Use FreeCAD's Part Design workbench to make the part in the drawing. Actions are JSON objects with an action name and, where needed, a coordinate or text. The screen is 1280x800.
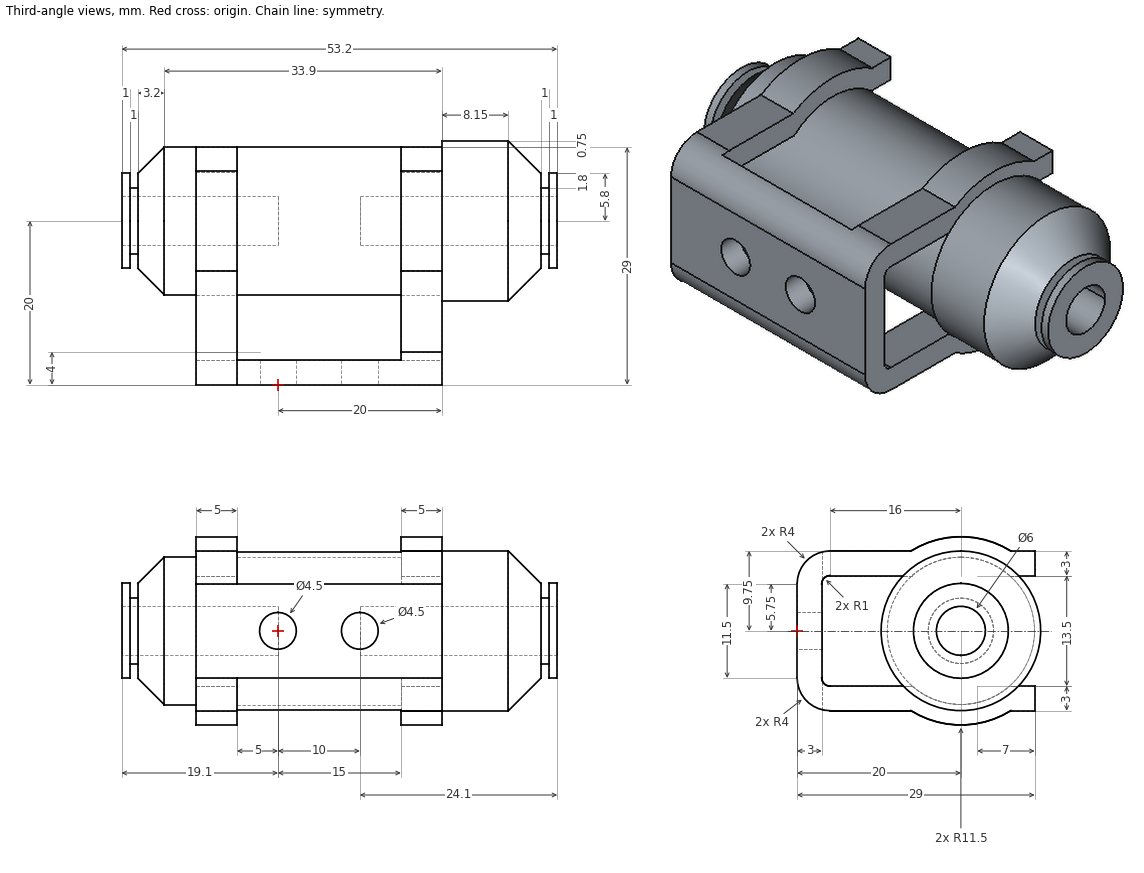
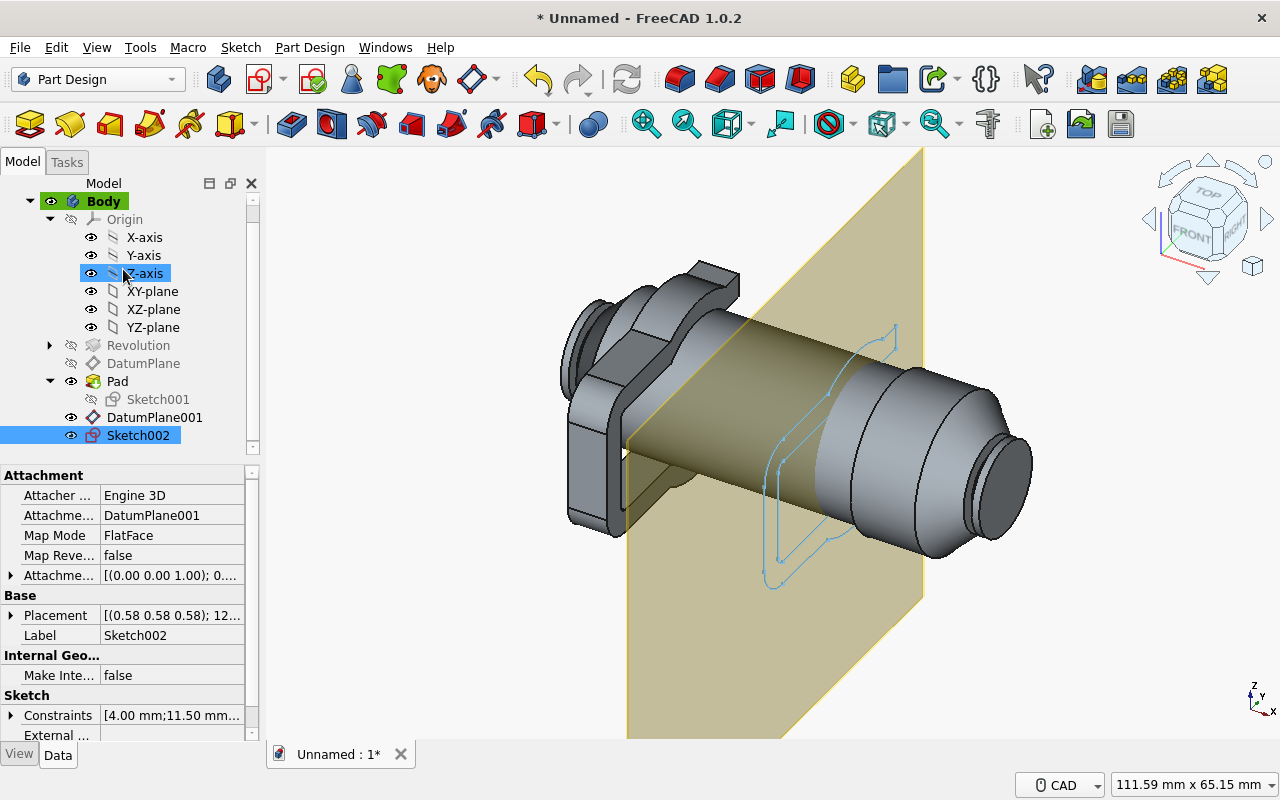
{"action": "left_click", "coordinate": [30, 124]}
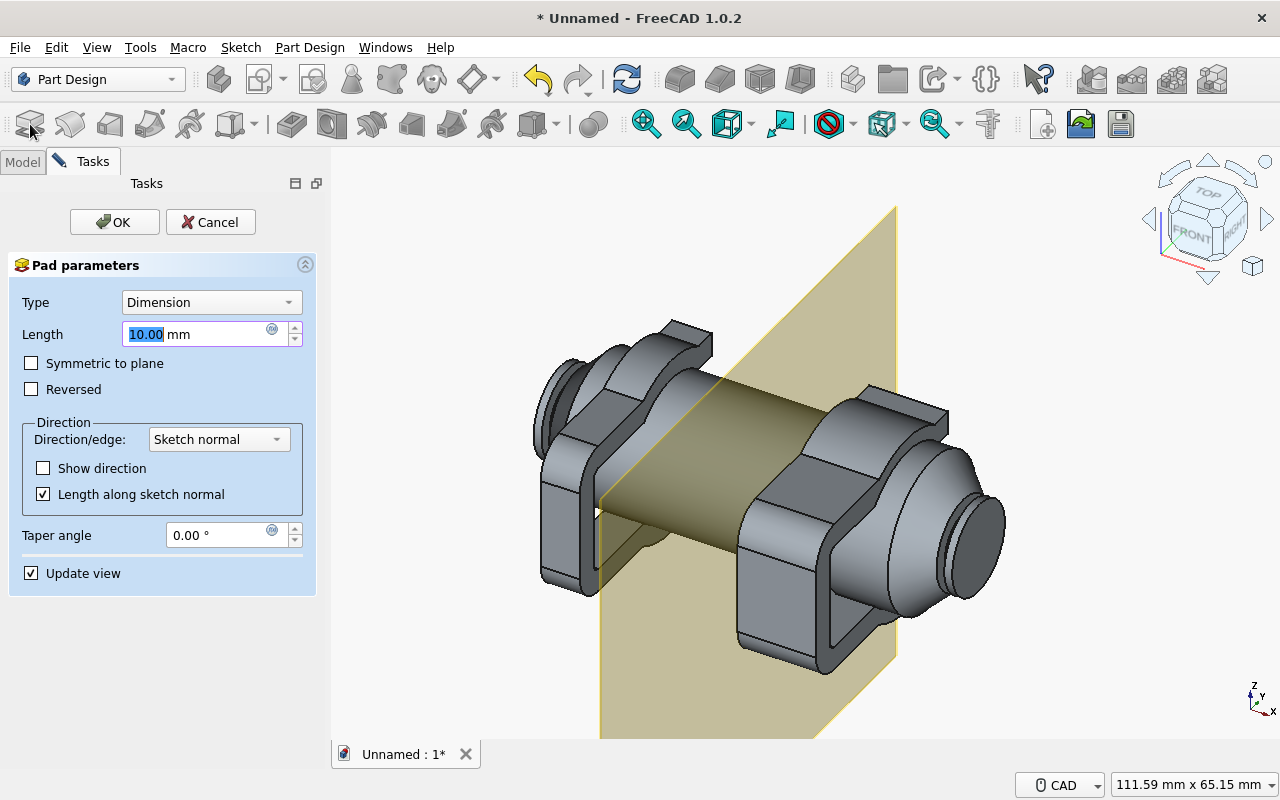
{"action": "type", "text": "5"}
{"action": "key", "text": "Tab"}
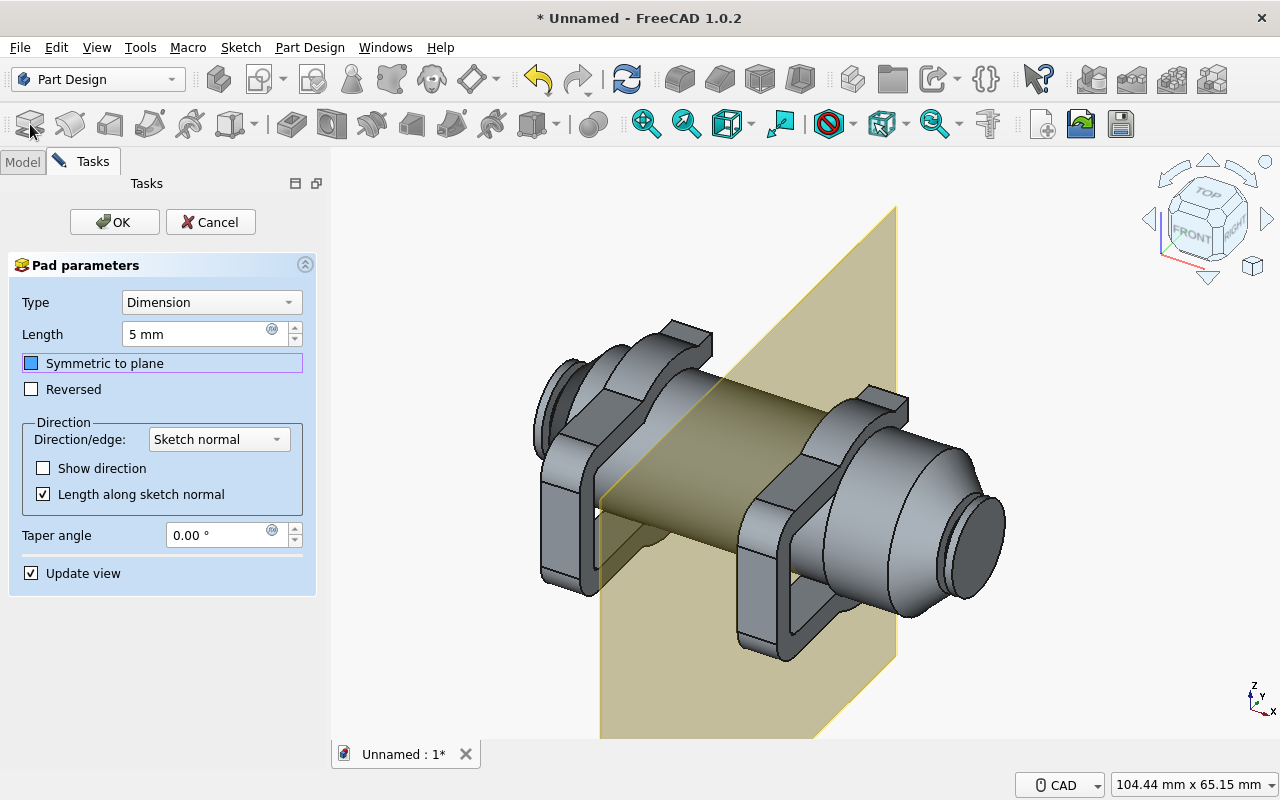
{"action": "left_click", "coordinate": [115, 222]}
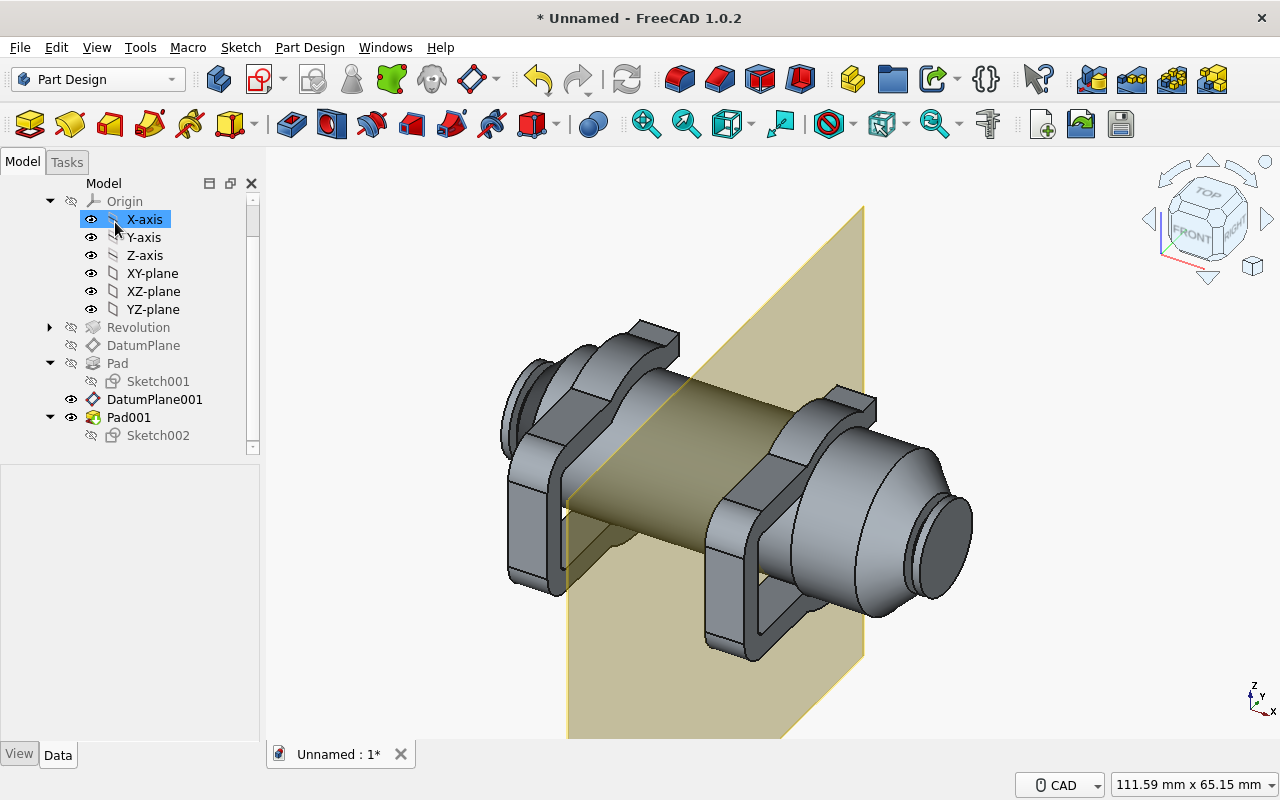
{"action": "left_click", "coordinate": [116, 399]}
{"action": "key", "text": "space"}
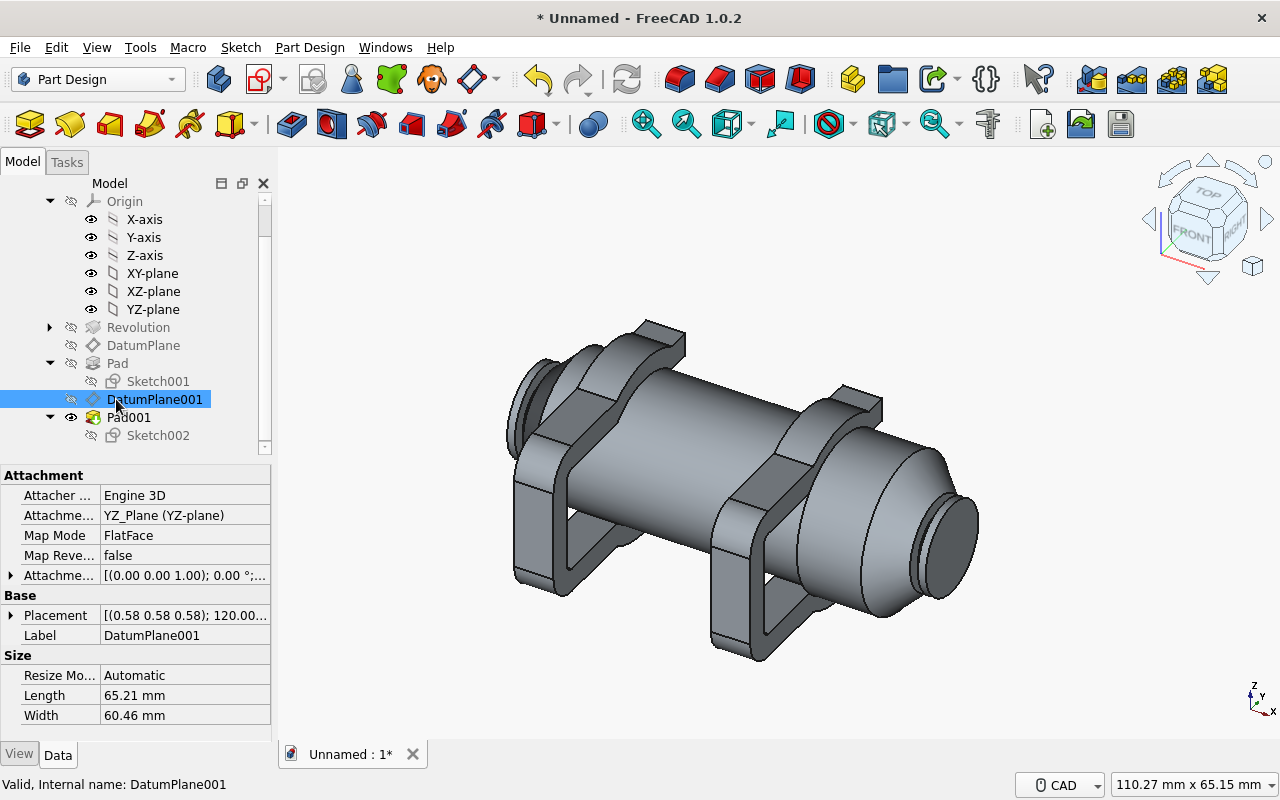
{"action": "left_click", "coordinate": [318, 699]}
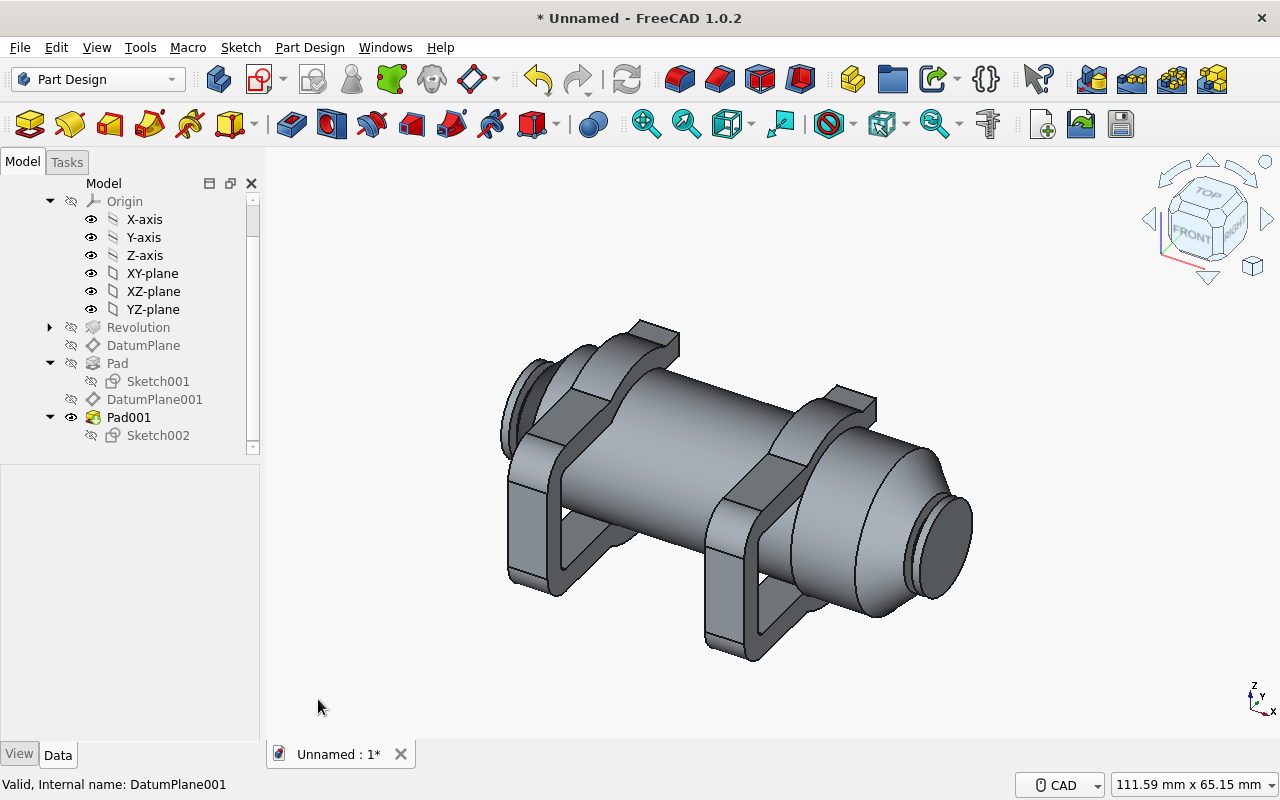
{"action": "left_click", "coordinate": [260, 80]}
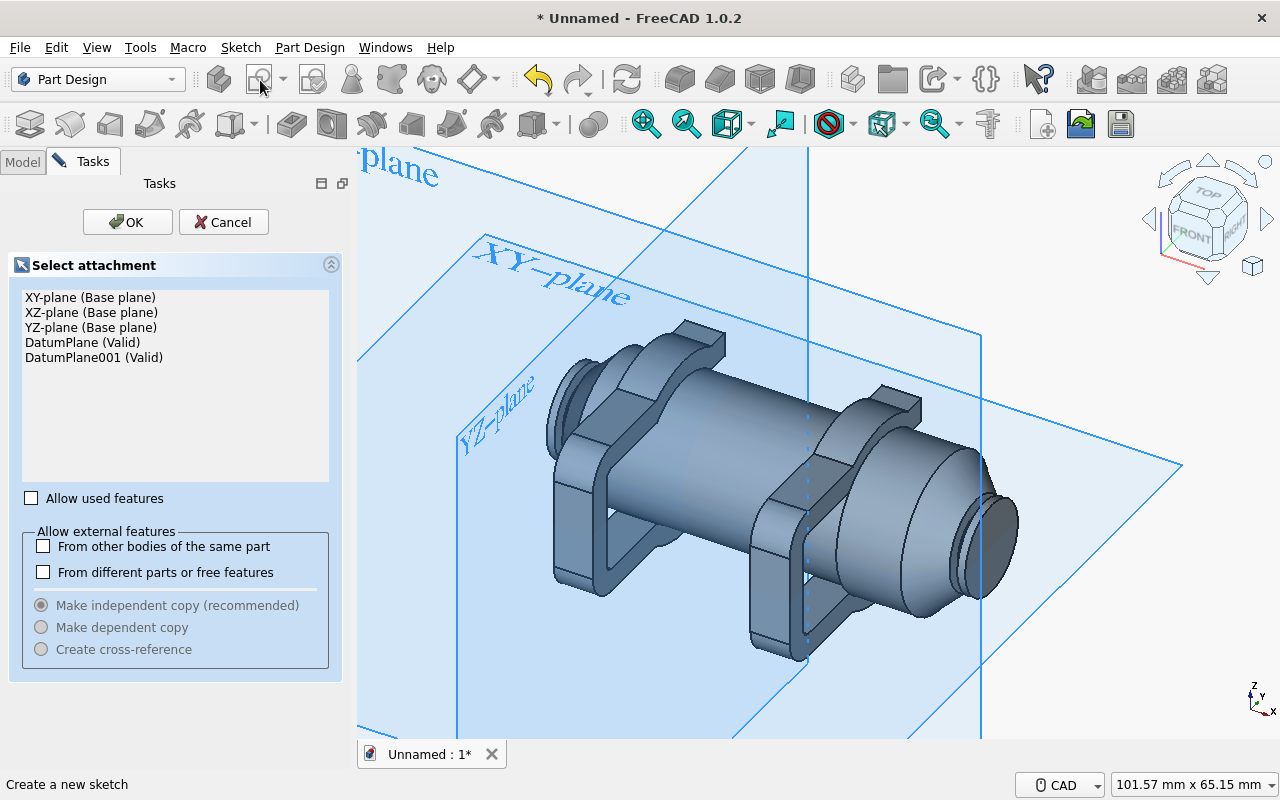
{"action": "left_click", "coordinate": [82, 328]}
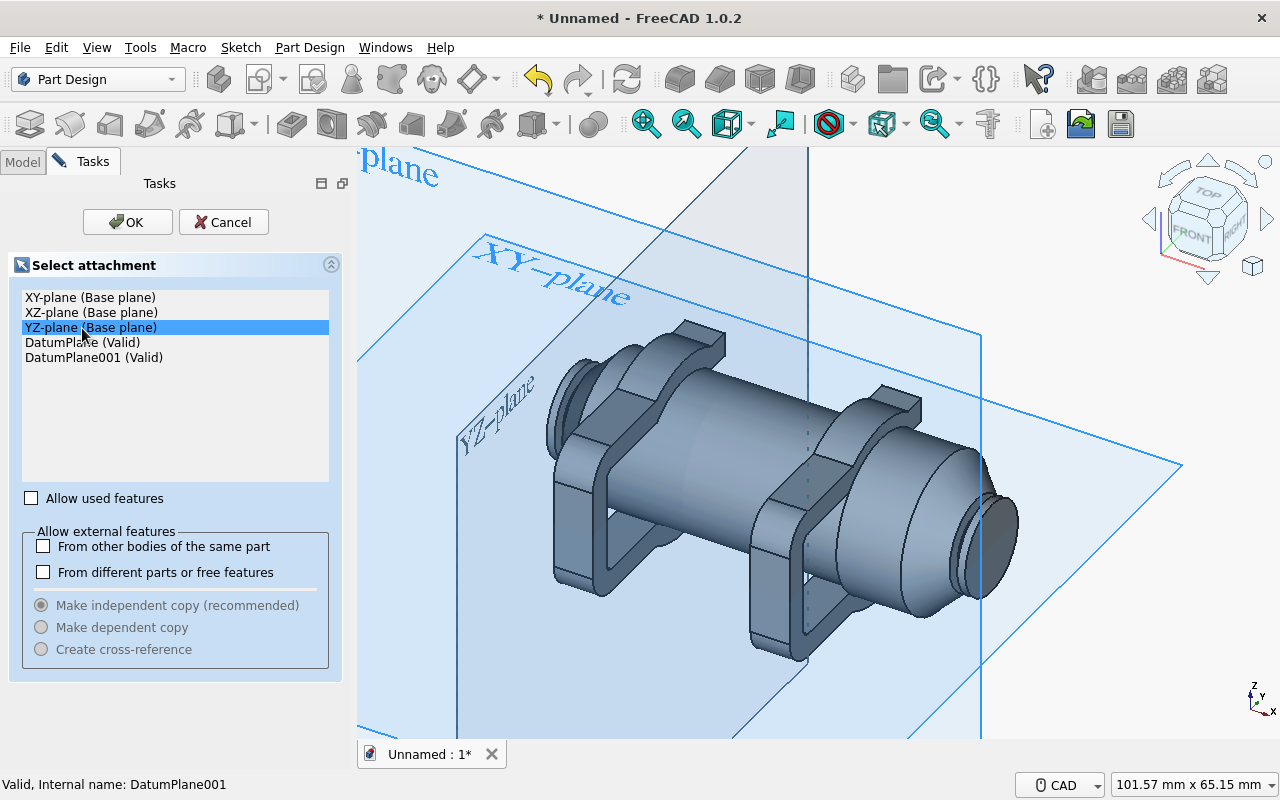
{"action": "left_click", "coordinate": [128, 222]}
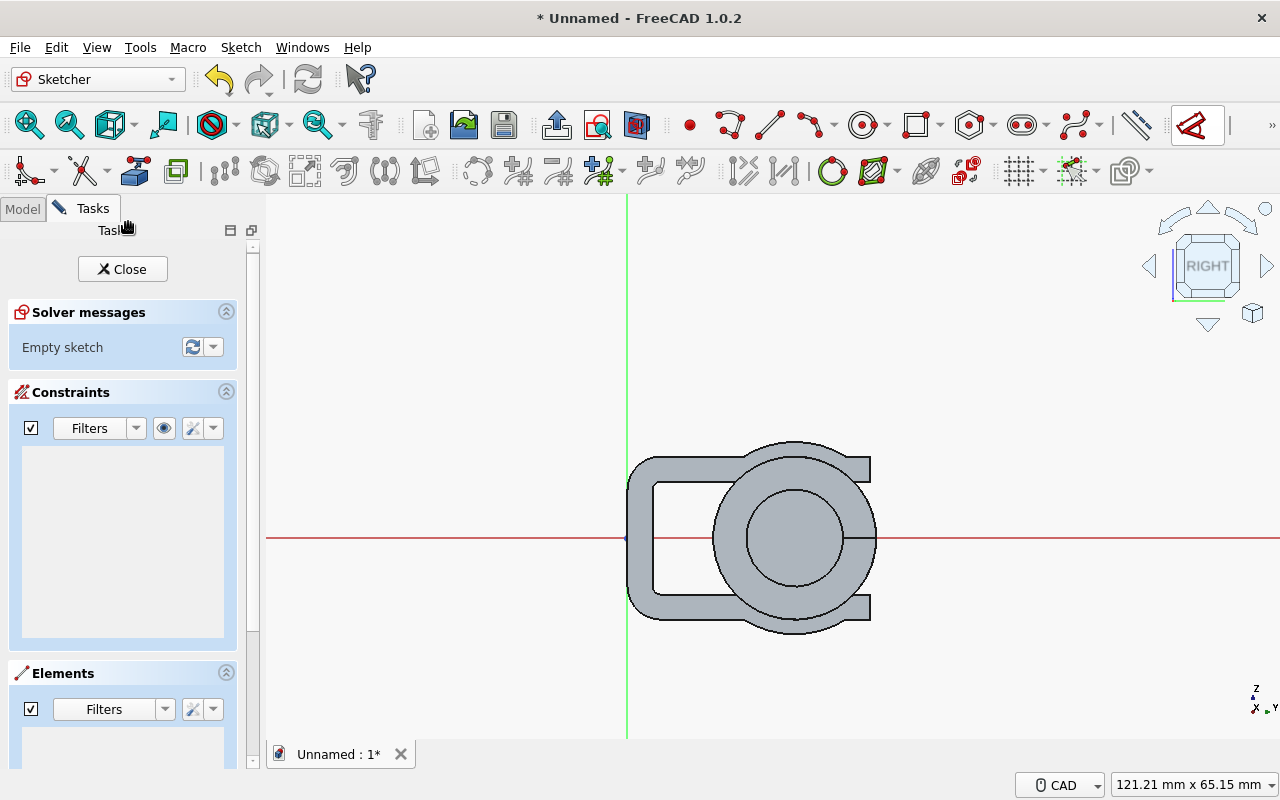
{"action": "left_click", "coordinate": [638, 126]}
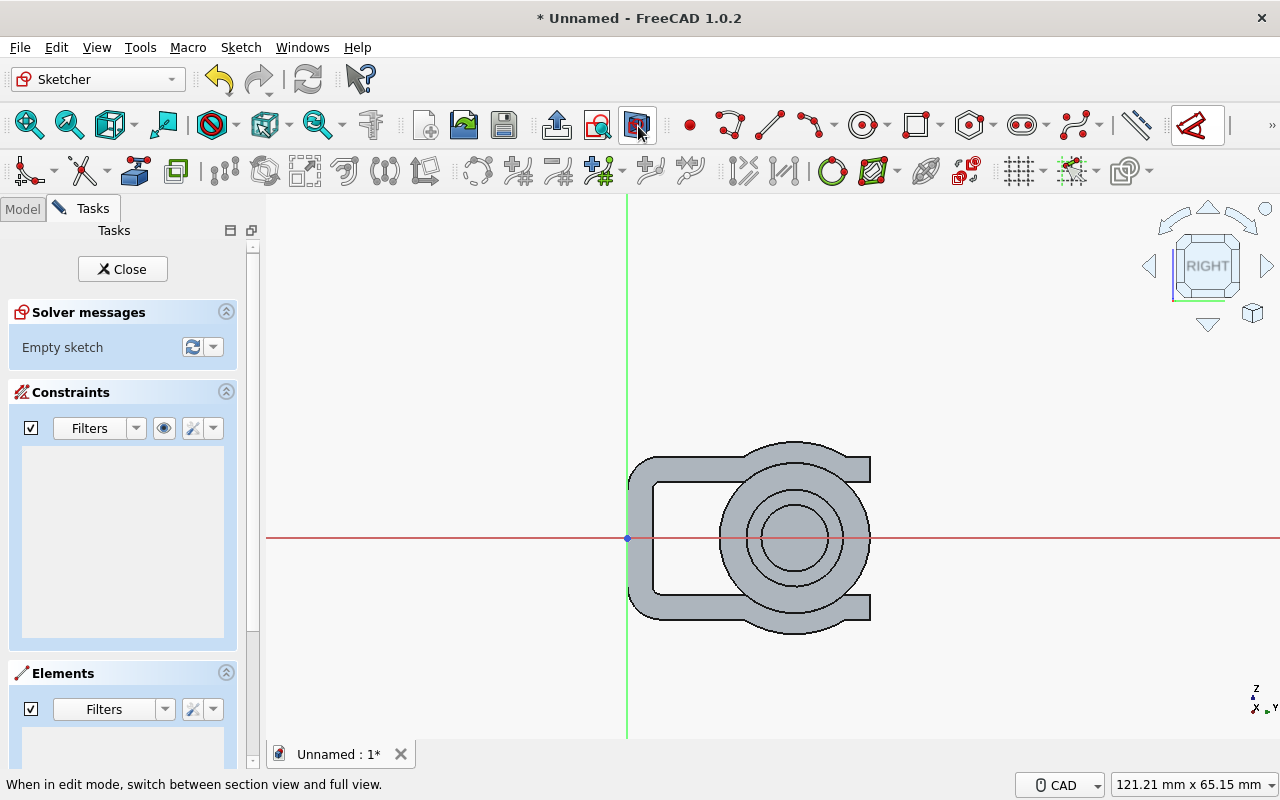
{"action": "scroll", "coordinate": [587, 597], "scroll_direction": "up", "scroll_amount": 4}